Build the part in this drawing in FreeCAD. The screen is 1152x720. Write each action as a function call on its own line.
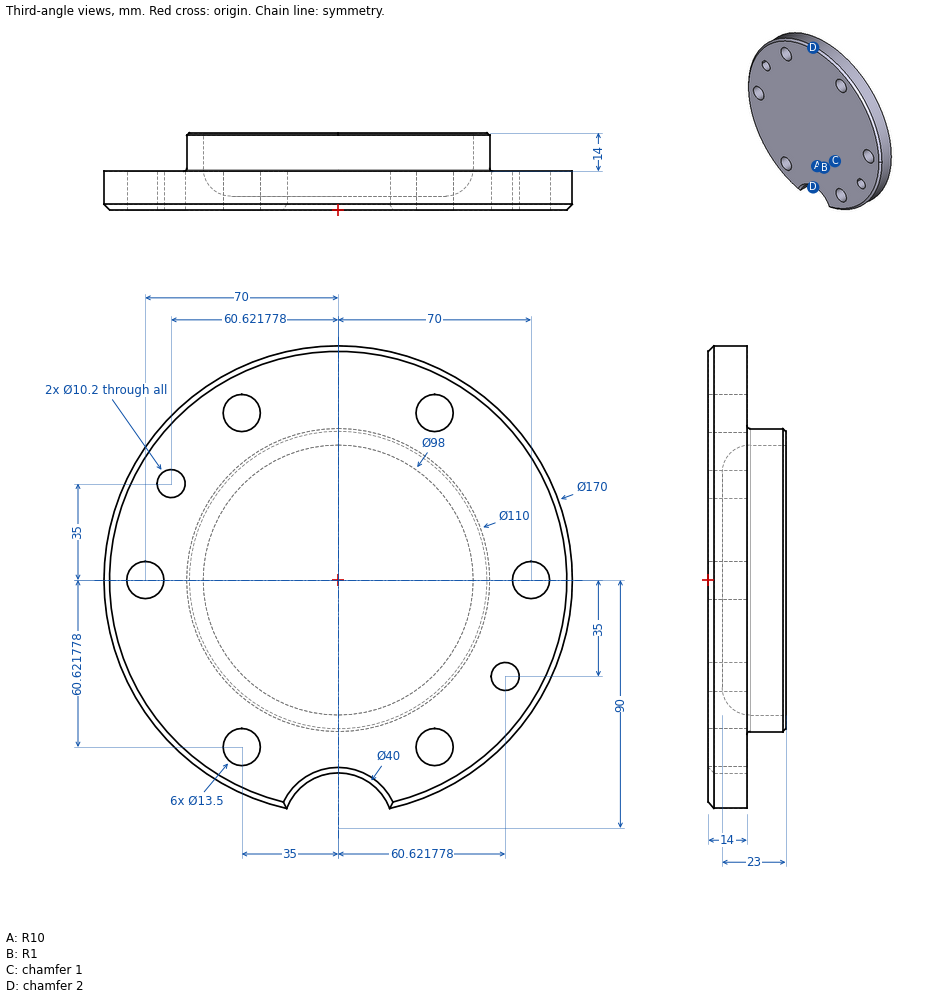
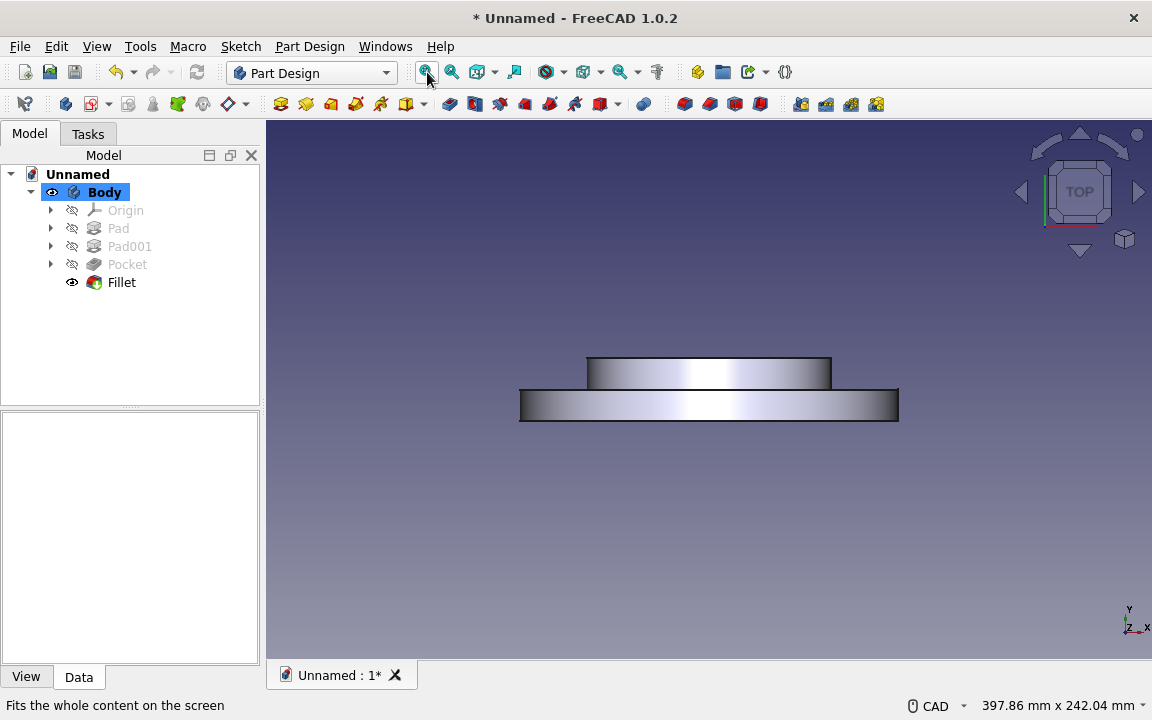
key(0)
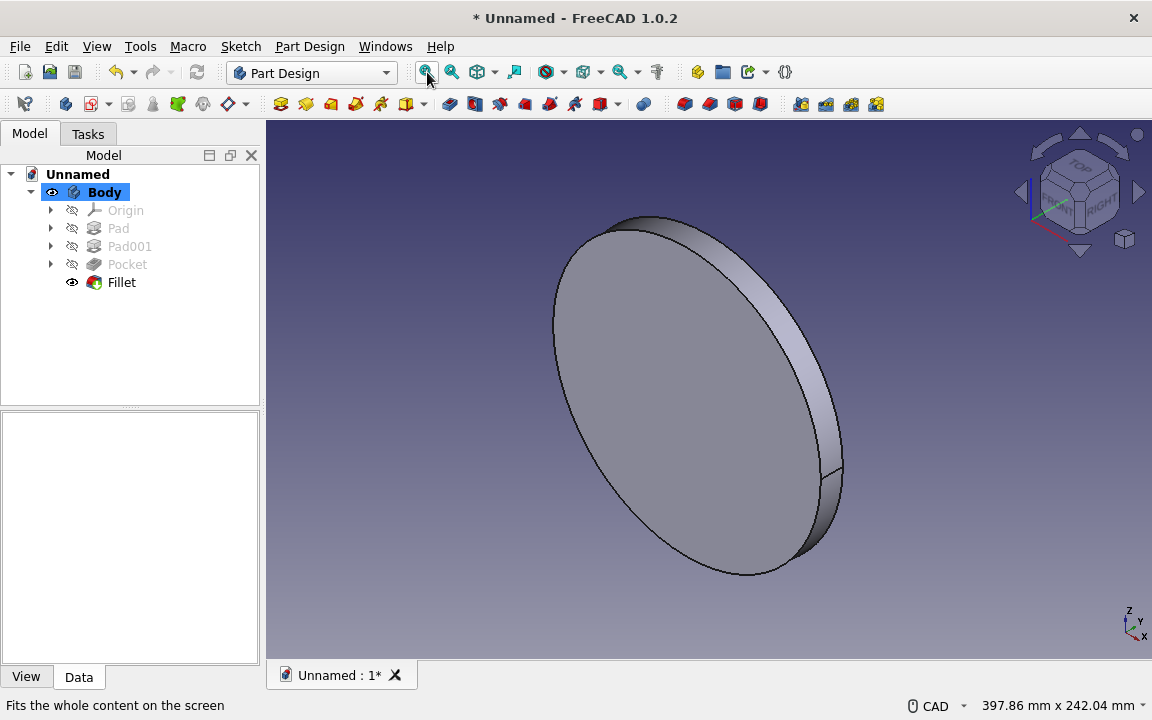
key(1)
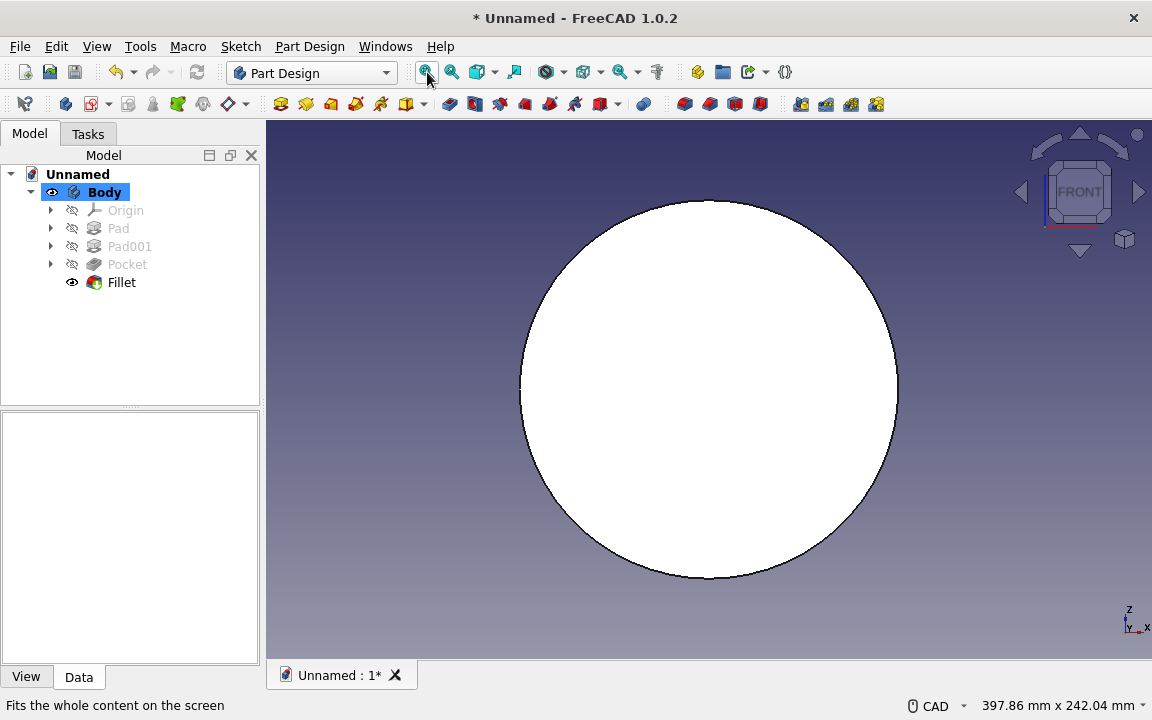
key(3)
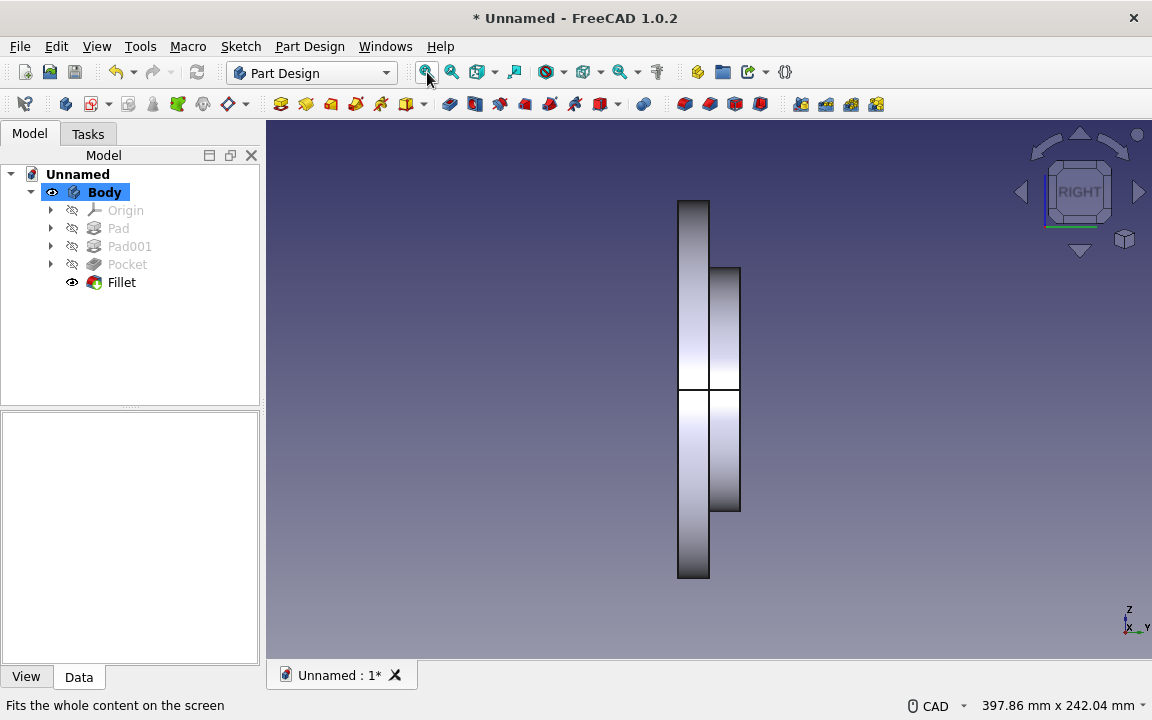
key(5)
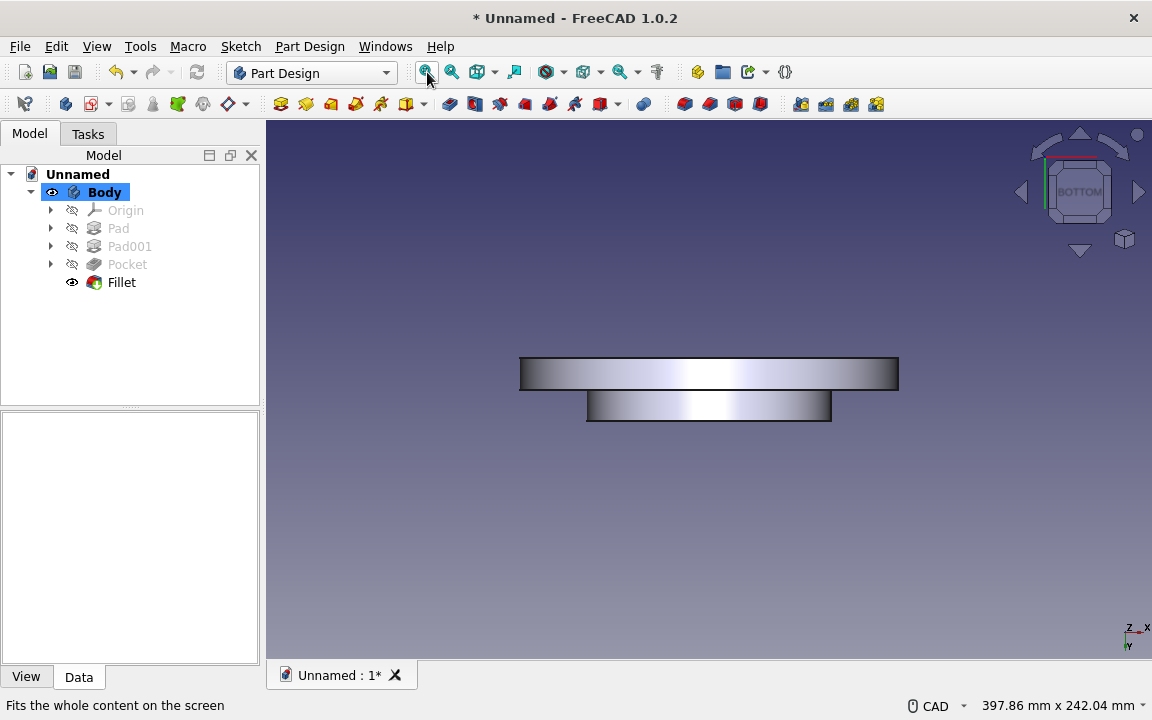
click(427, 72)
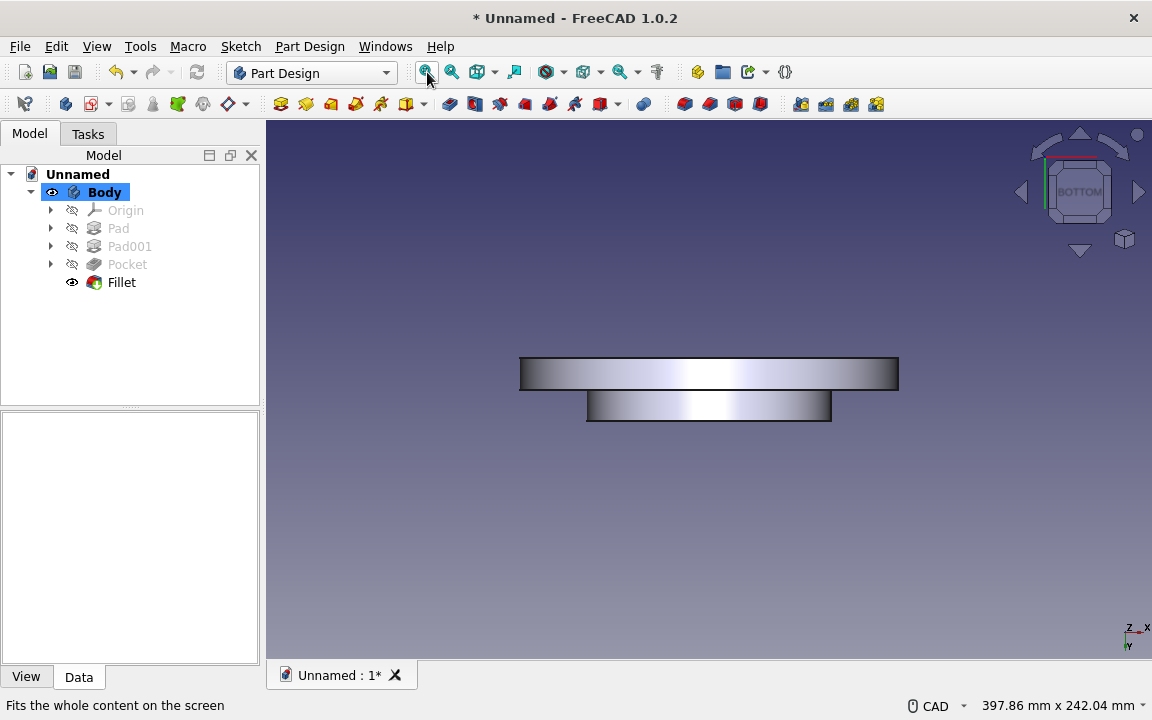
key(4)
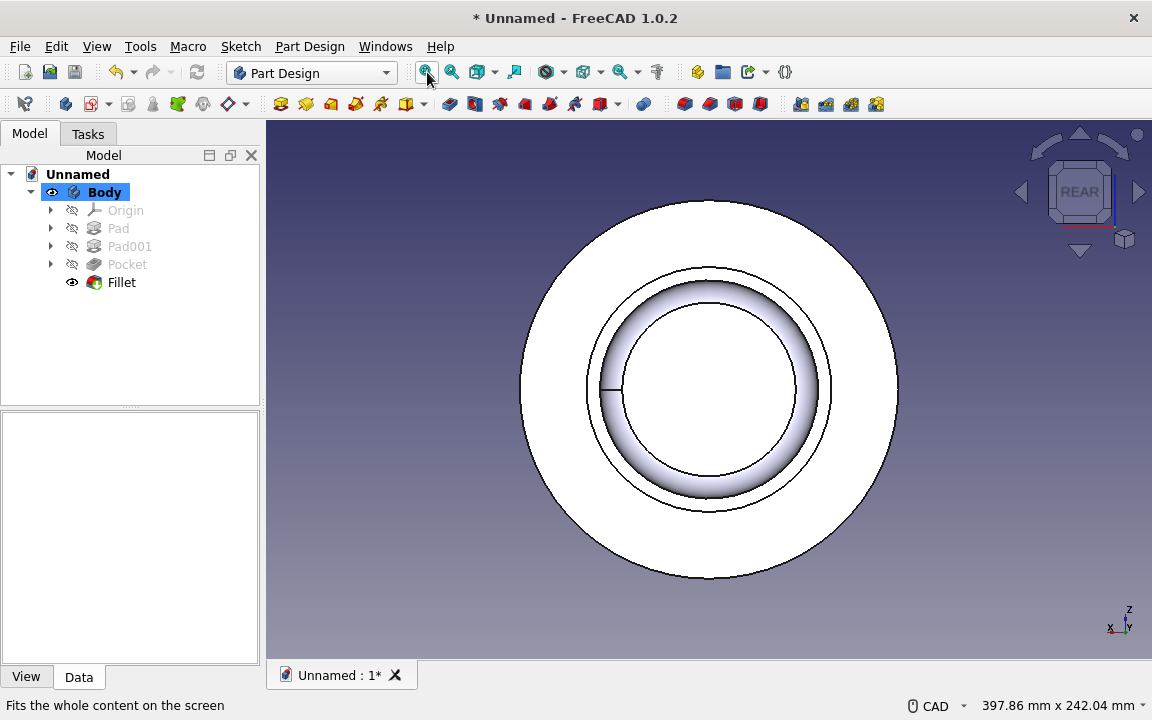
key(6)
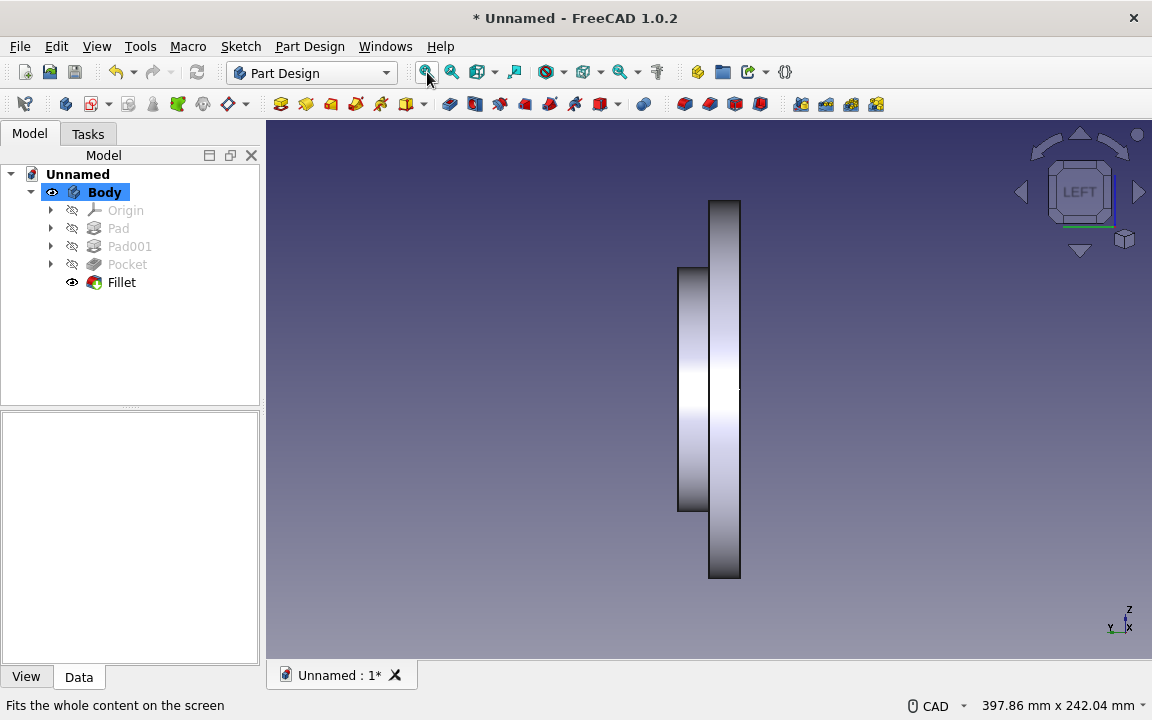
key(v)
key(3)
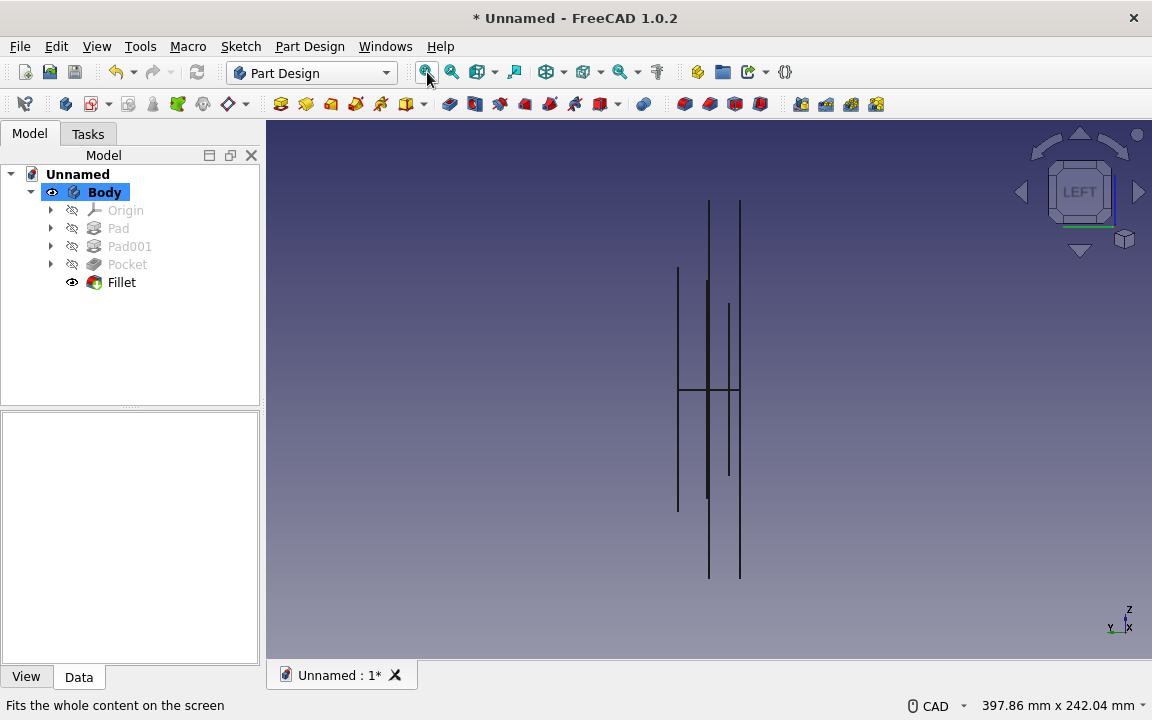
key(0)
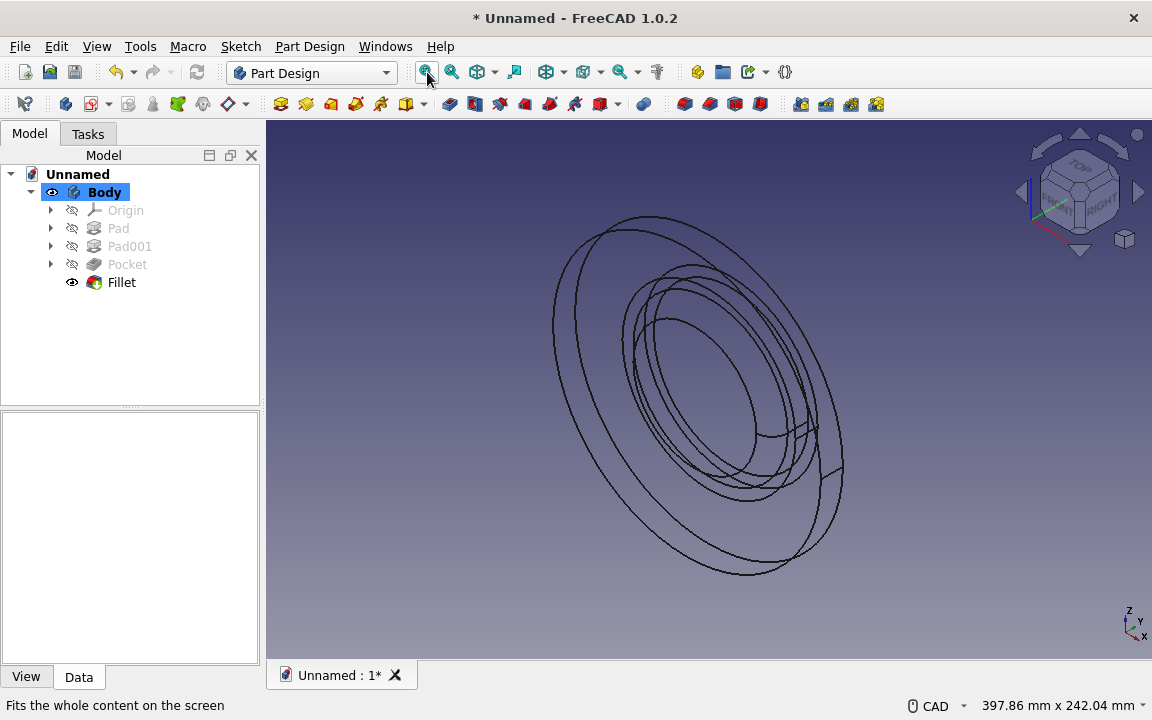
click(622, 338)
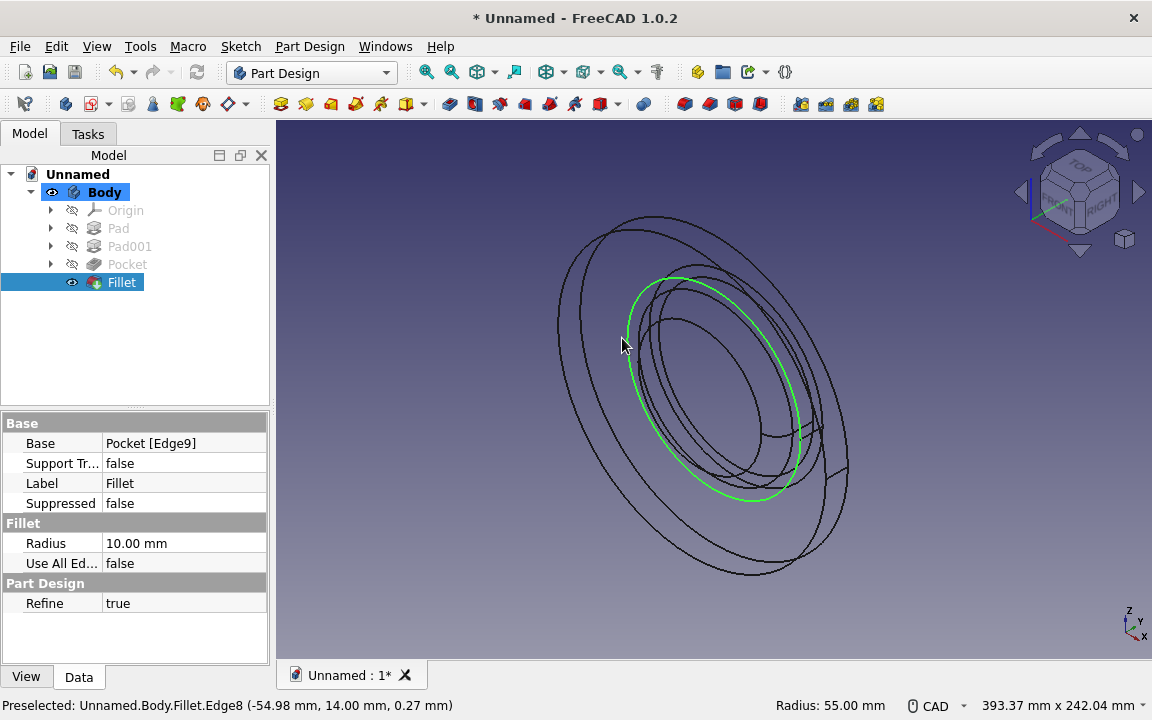
key(v)
key(1)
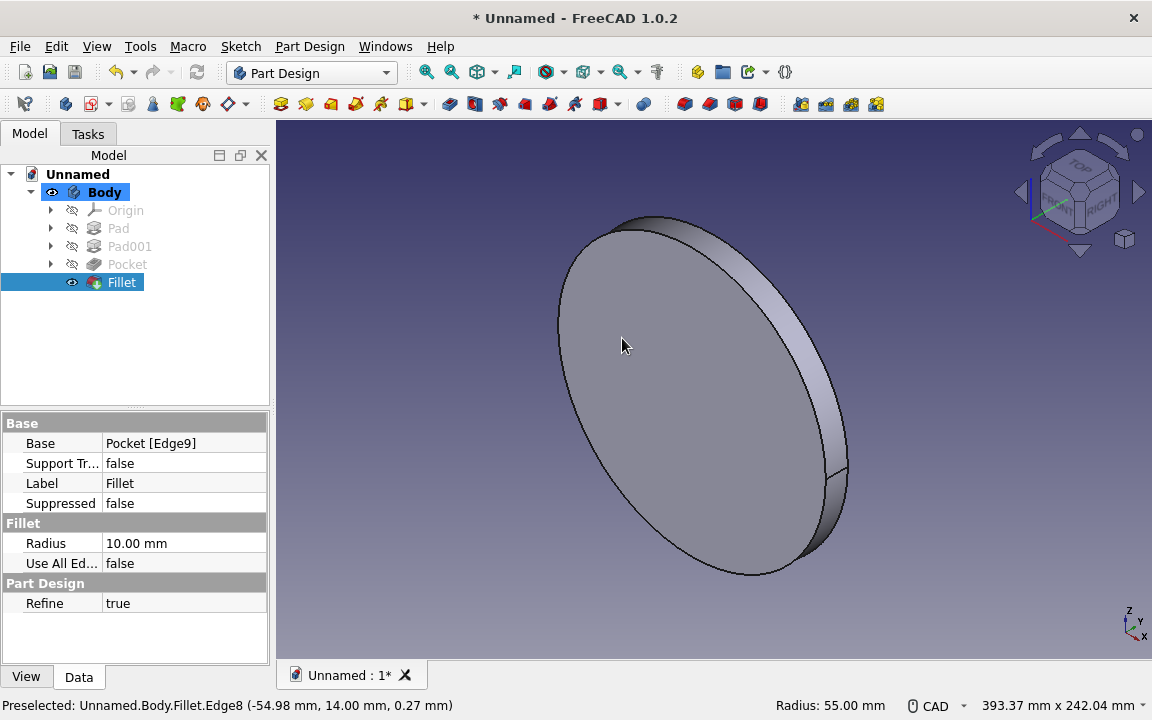
click(685, 104)